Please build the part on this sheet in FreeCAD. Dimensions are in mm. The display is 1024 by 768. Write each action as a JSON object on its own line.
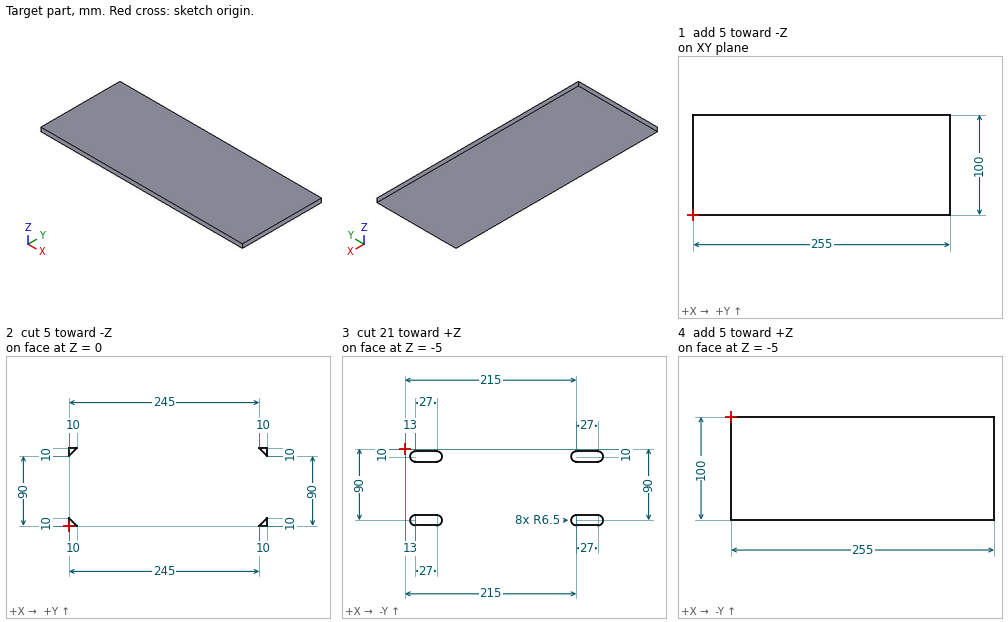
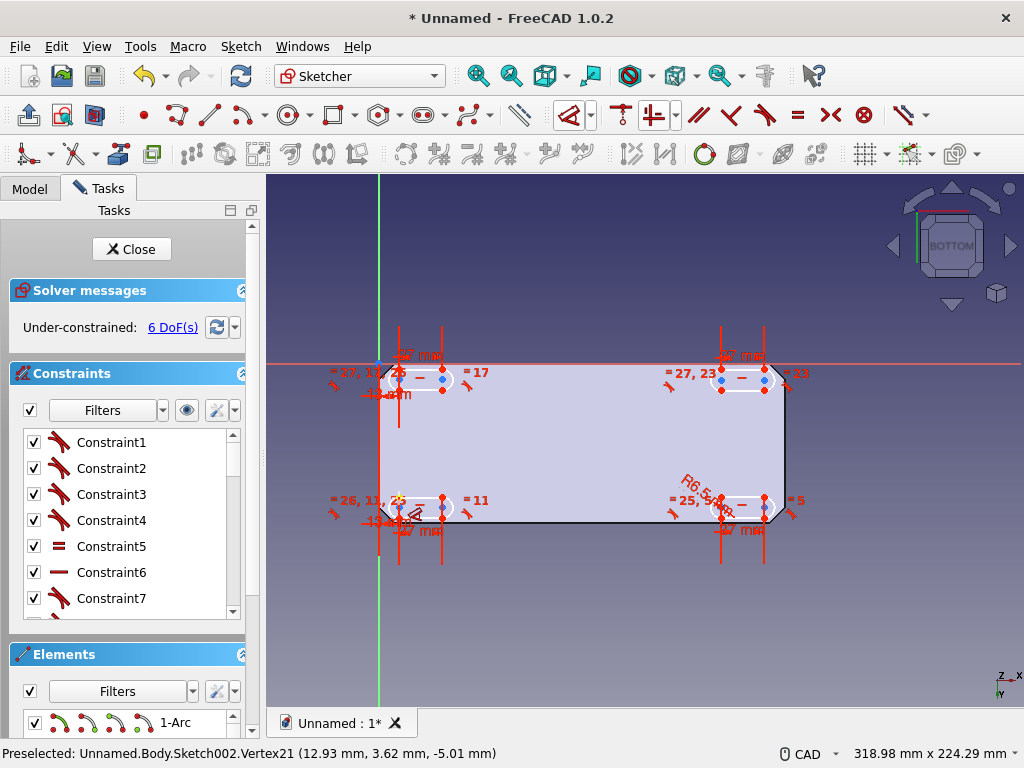
{"action": "left_click", "coordinate": [721, 508]}
{"action": "left_click", "coordinate": [345, 436]}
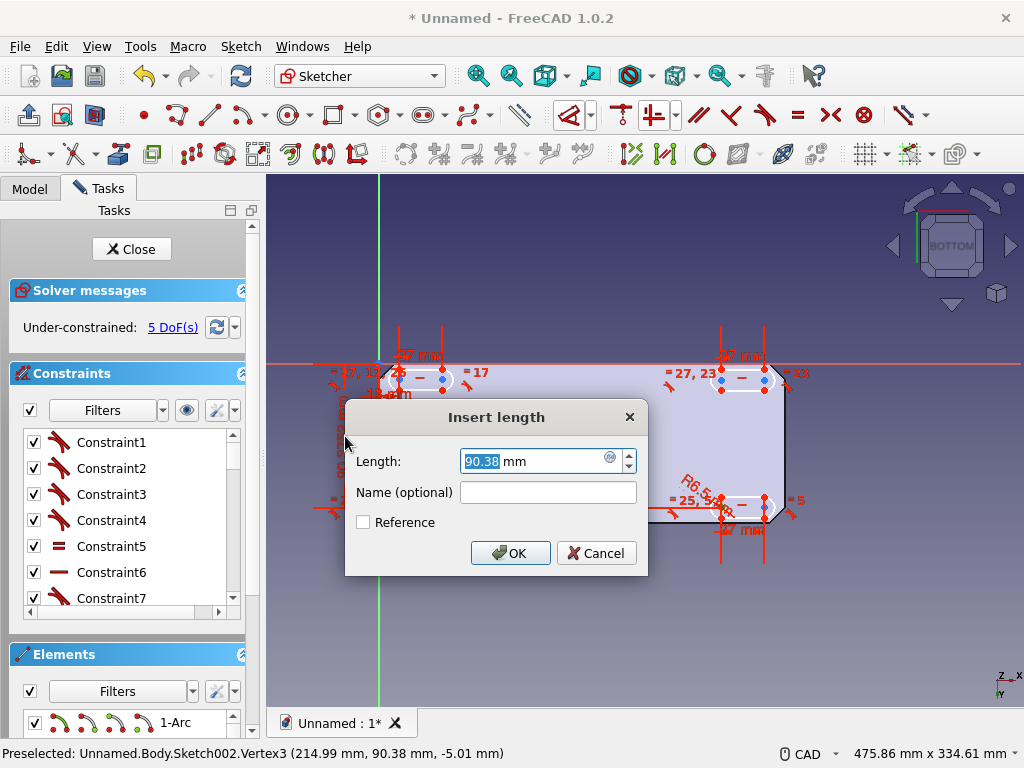
{"action": "type", "text": "90"}
{"action": "key", "text": "Return"}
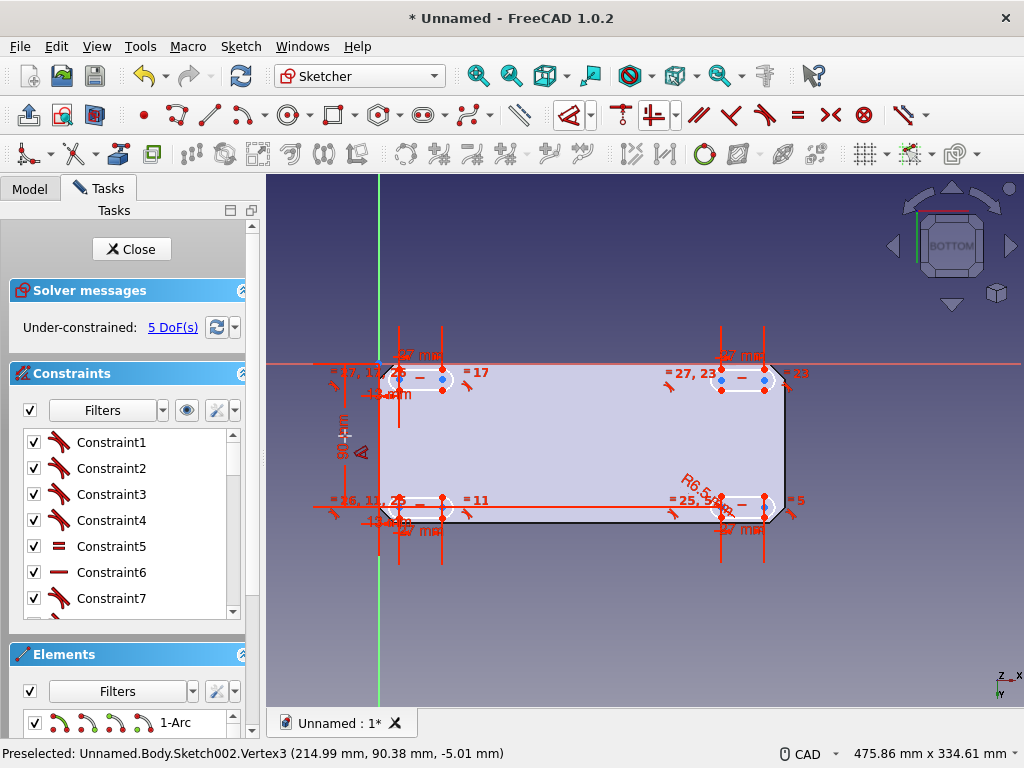
{"action": "left_click", "coordinate": [399, 508]}
{"action": "left_click", "coordinate": [345, 469]}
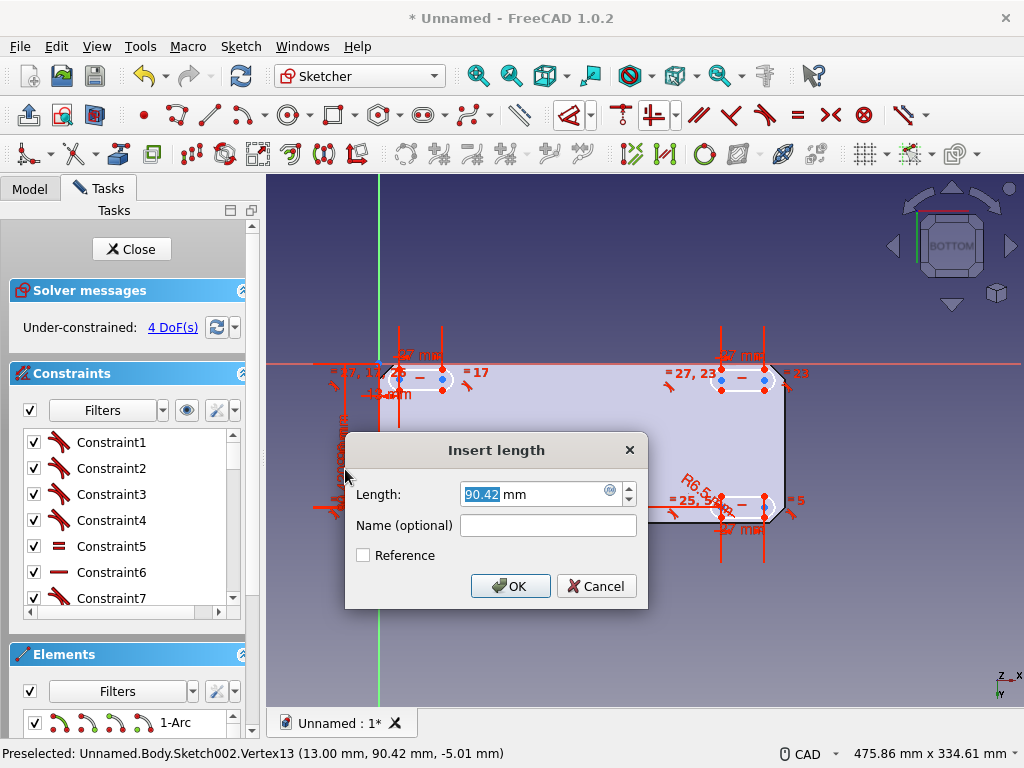
{"action": "type", "text": "90"}
{"action": "key", "text": "Return"}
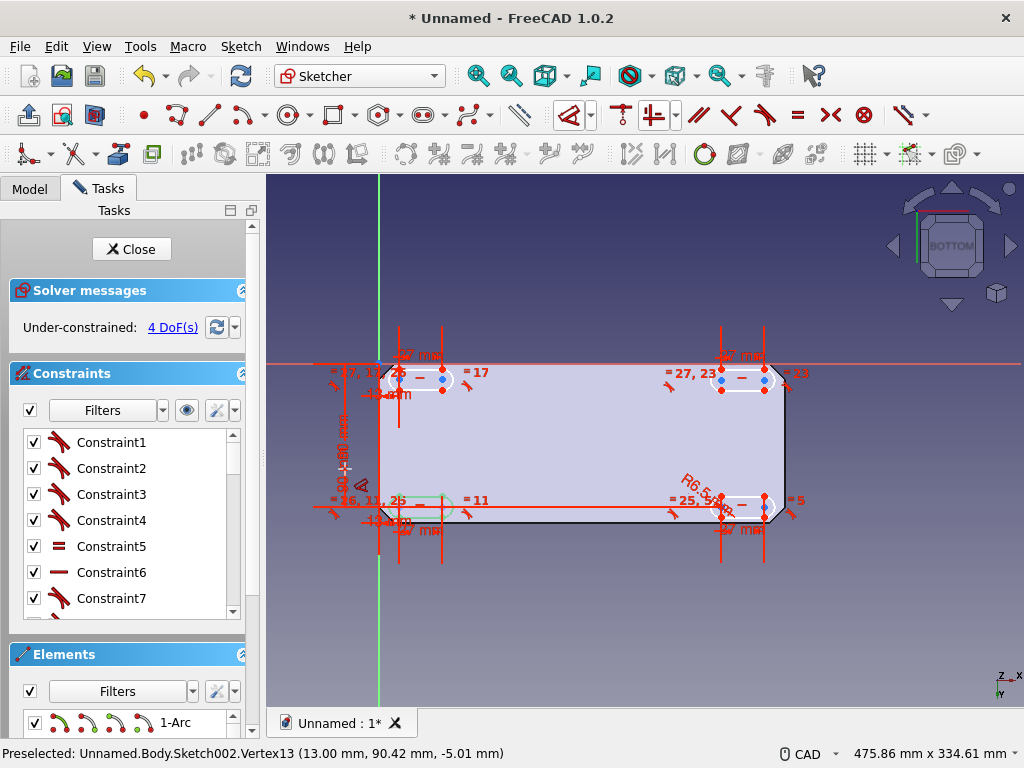
{"action": "scroll", "coordinate": [399, 380], "scroll_direction": "up", "scroll_amount": 5}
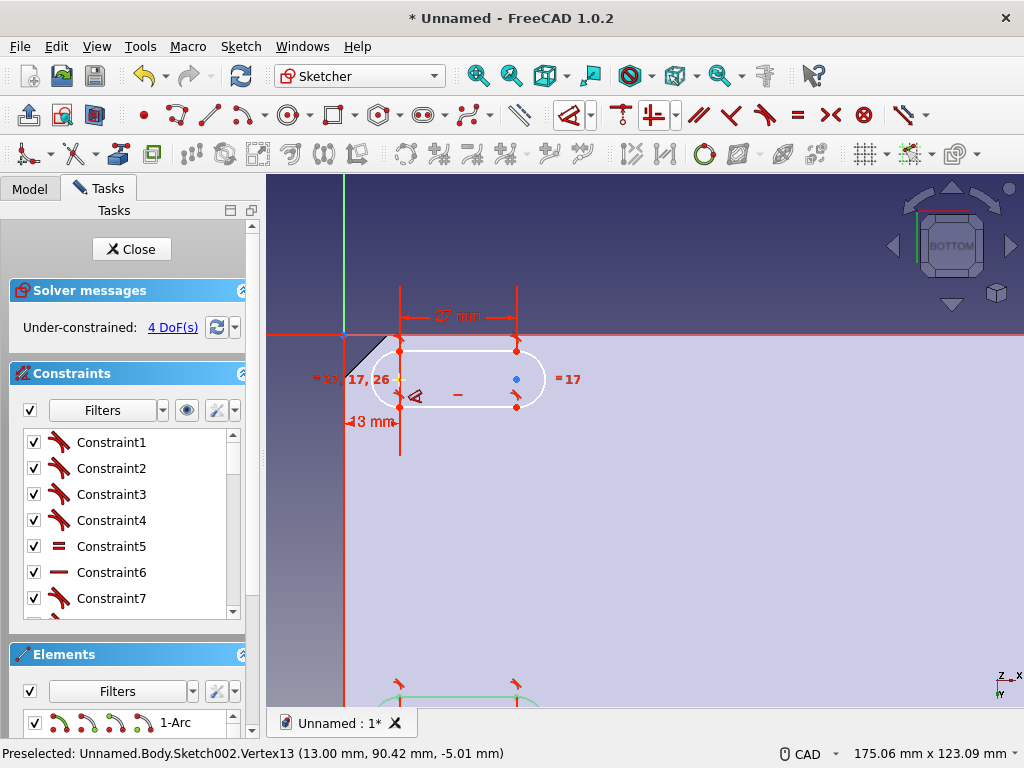
{"action": "left_click", "coordinate": [400, 379]}
{"action": "left_click", "coordinate": [310, 357]}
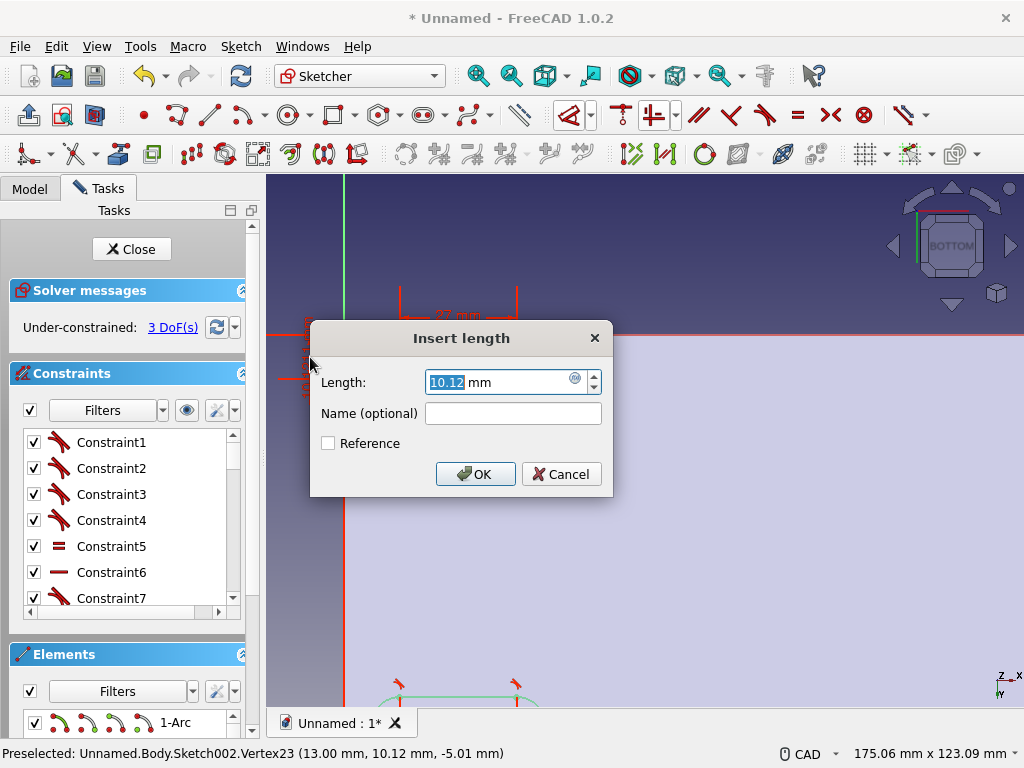
{"action": "type", "text": "10"}
{"action": "key", "text": "Return"}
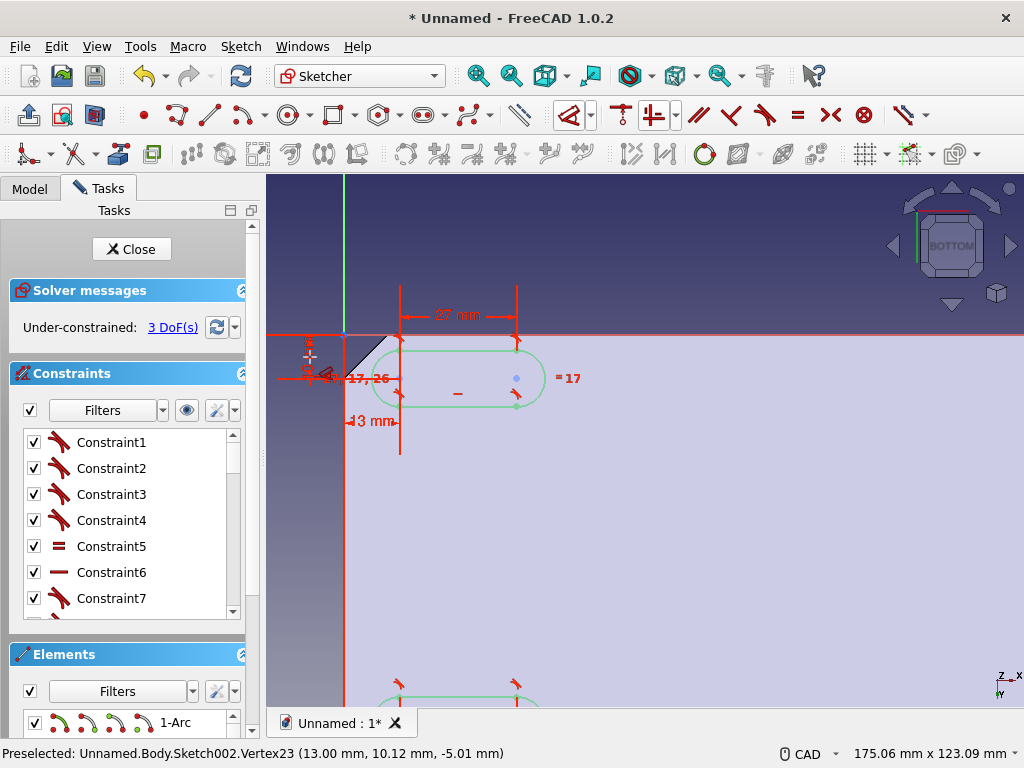
{"action": "scroll", "coordinate": [399, 380], "scroll_direction": "down", "scroll_amount": 5}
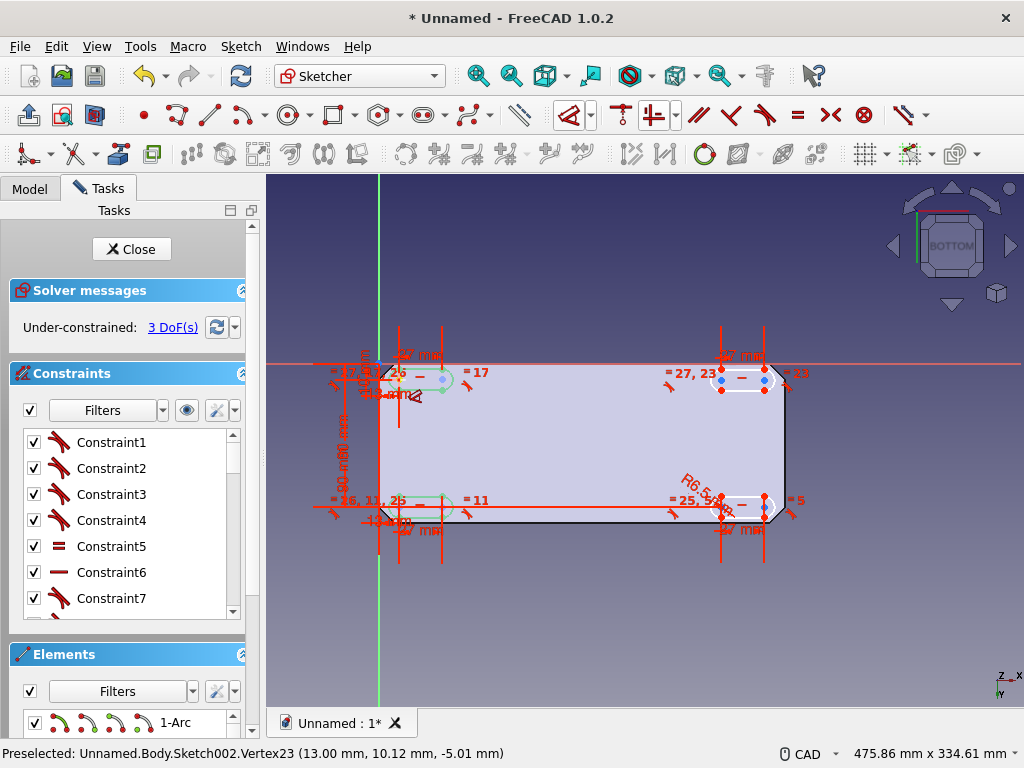
{"action": "scroll", "coordinate": [721, 380], "scroll_direction": "up", "scroll_amount": 5}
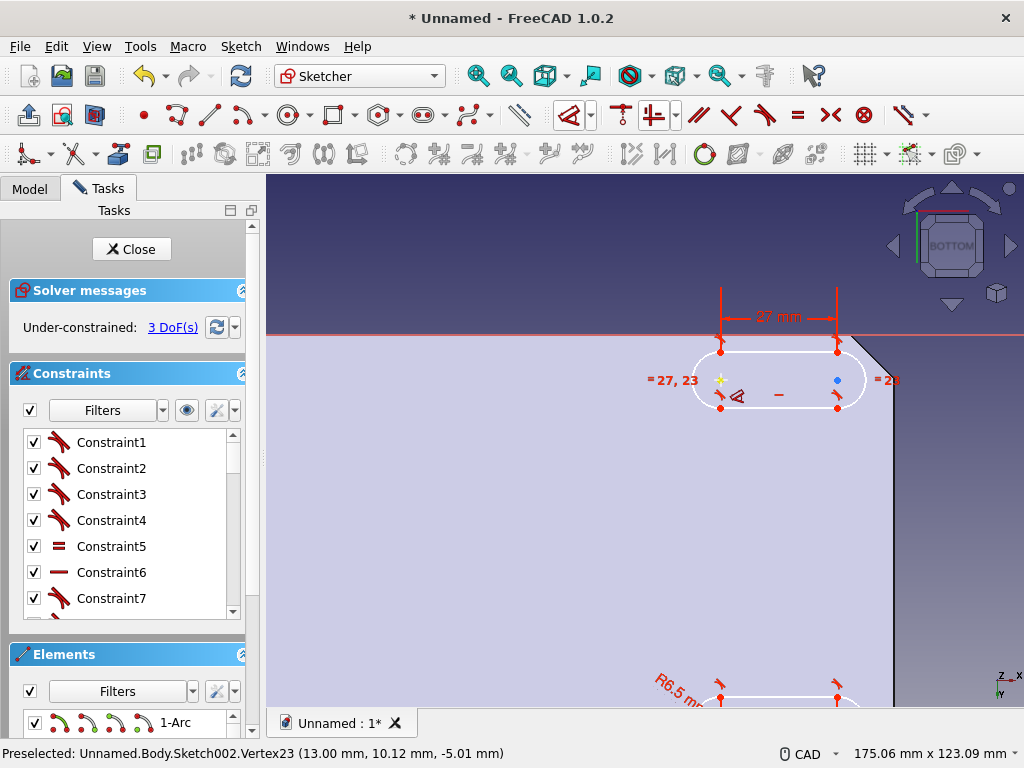
{"action": "left_click", "coordinate": [721, 380]}
{"action": "left_click", "coordinate": [755, 368]}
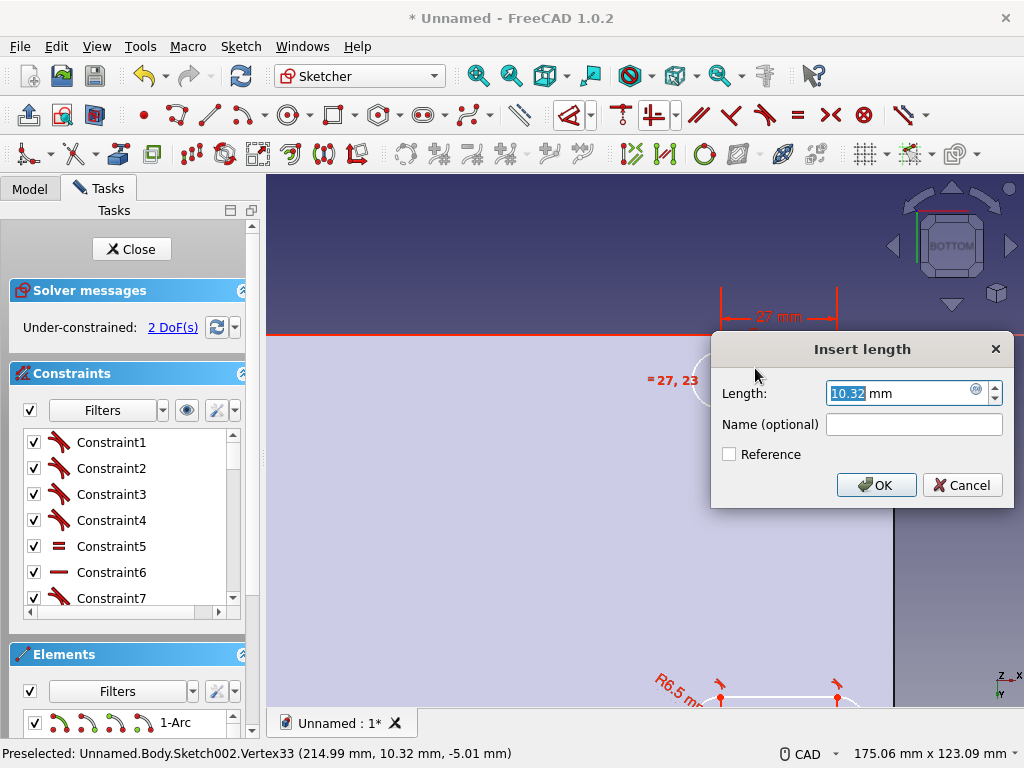
{"action": "type", "text": "10"}
{"action": "key", "text": "Return"}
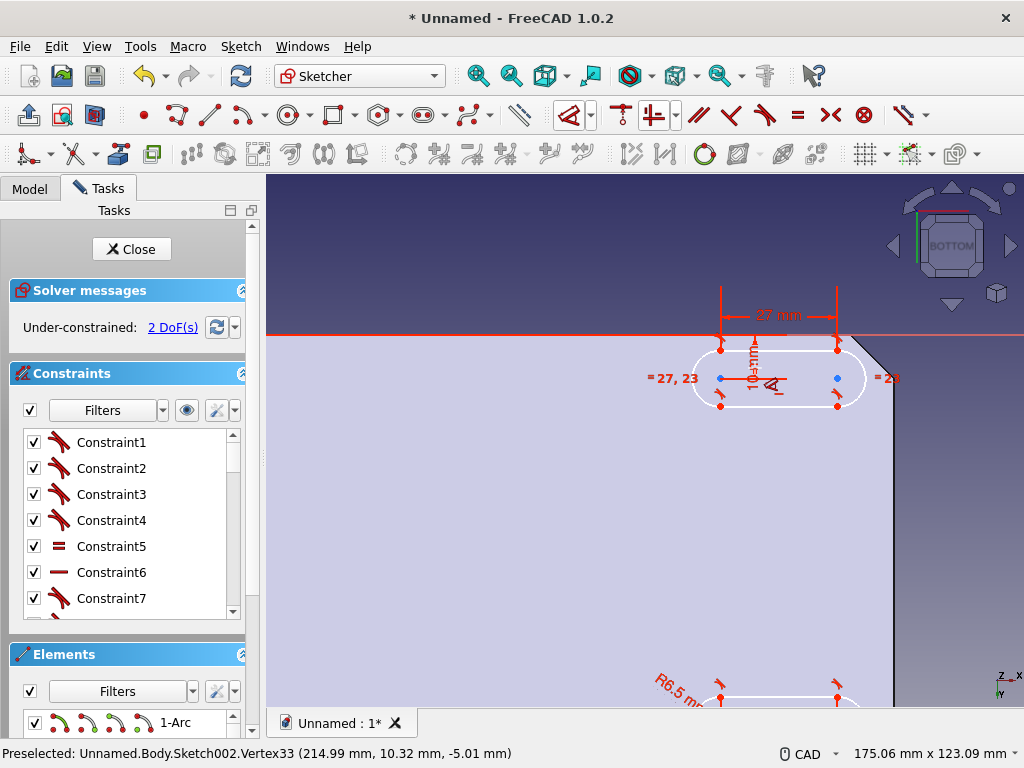
{"action": "scroll", "coordinate": [721, 380], "scroll_direction": "down", "scroll_amount": 5}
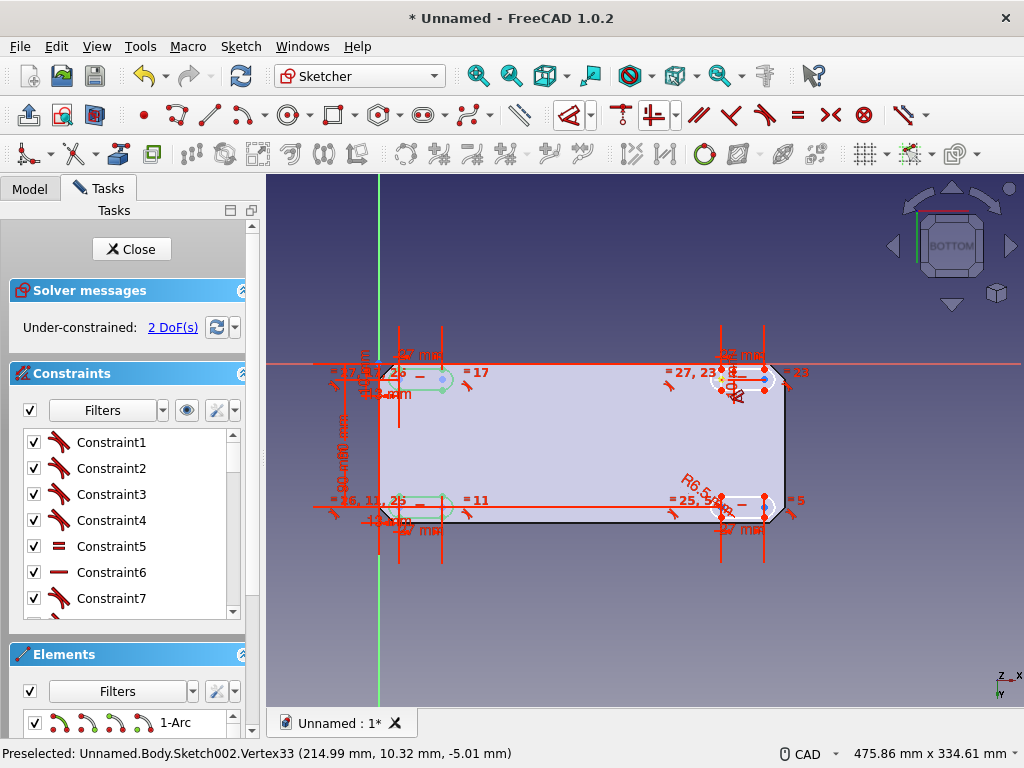
{"action": "left_click", "coordinate": [721, 497]}
{"action": "left_click", "coordinate": [550, 330]}